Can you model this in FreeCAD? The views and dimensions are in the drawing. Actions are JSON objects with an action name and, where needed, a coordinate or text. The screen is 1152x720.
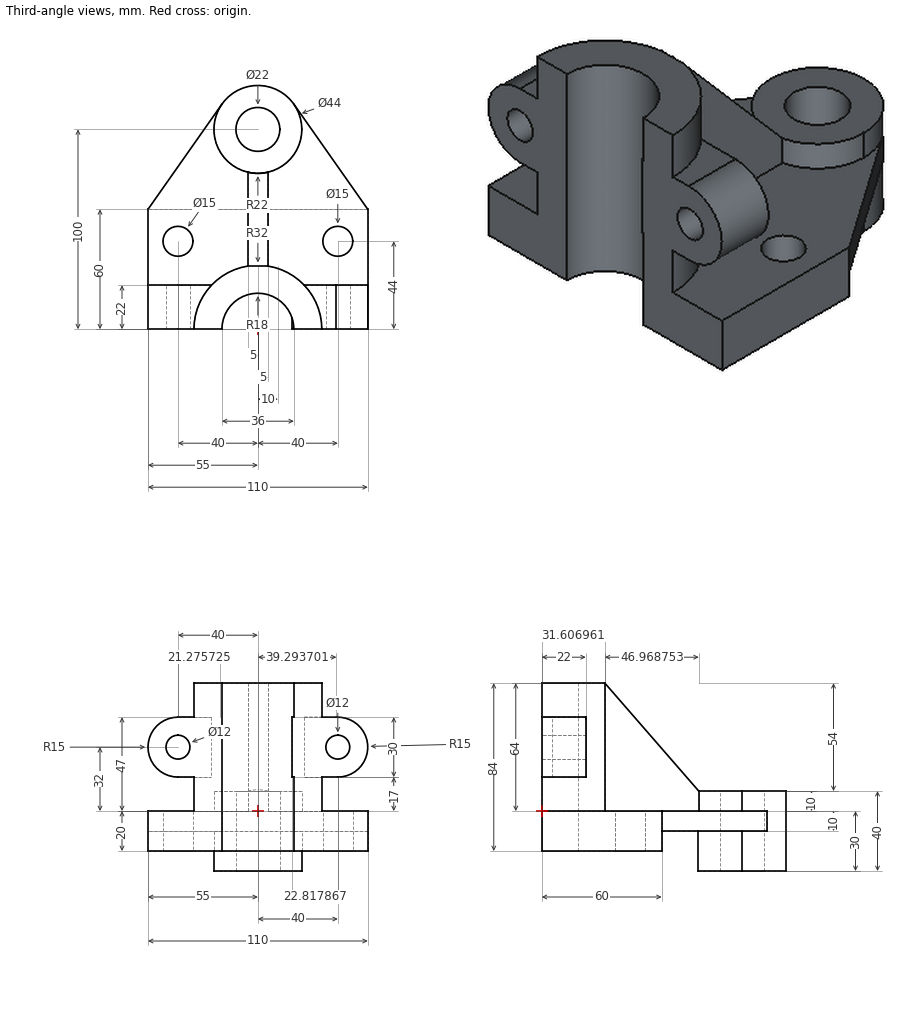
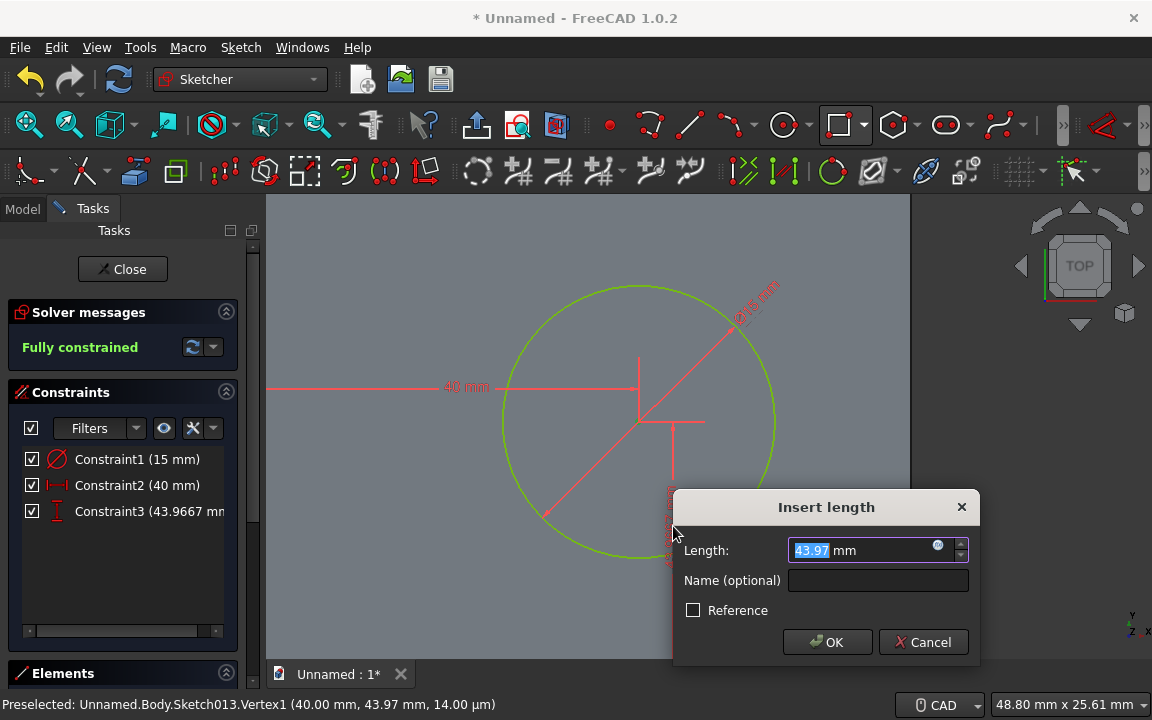
{"action": "type", "text": "44"}
{"action": "key", "text": "Return"}
{"action": "key", "text": "Escape"}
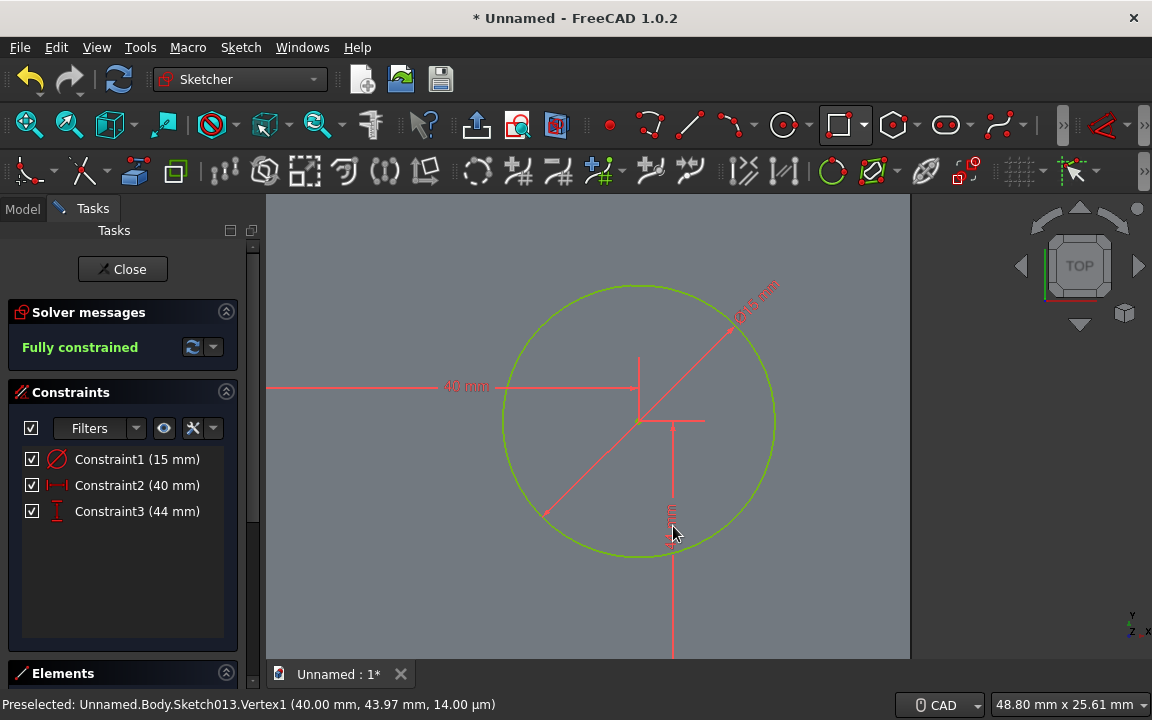
{"action": "left_click", "coordinate": [123, 269]}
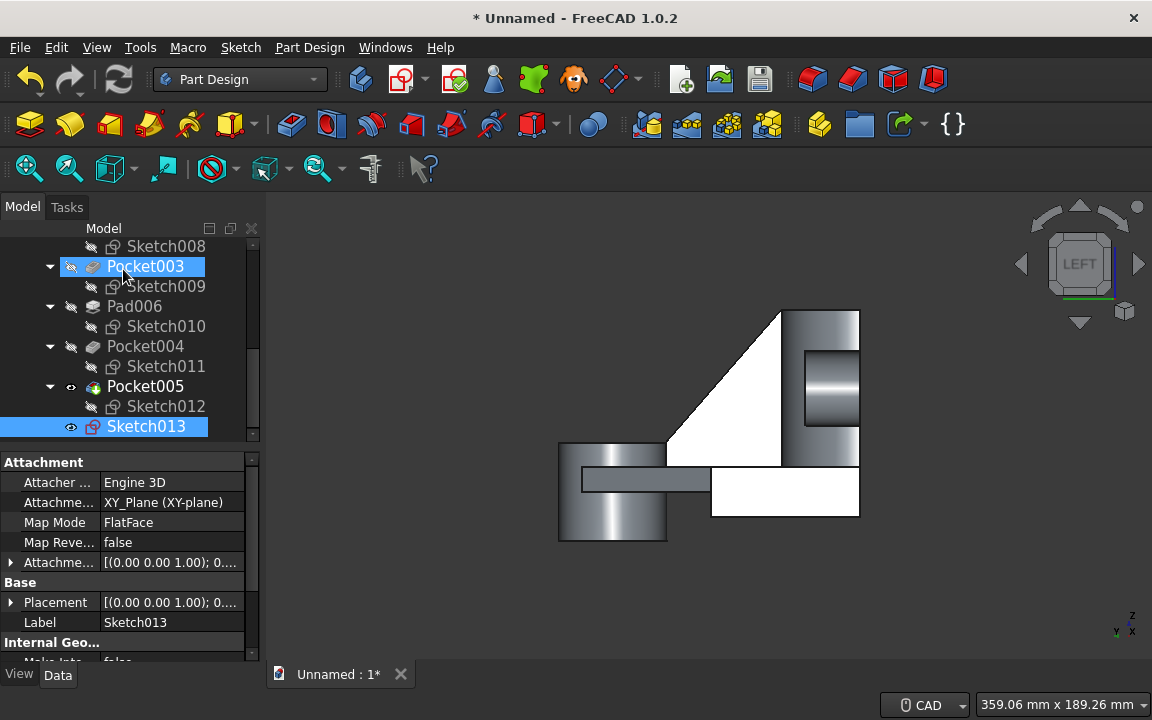
{"action": "left_click", "coordinate": [292, 124]}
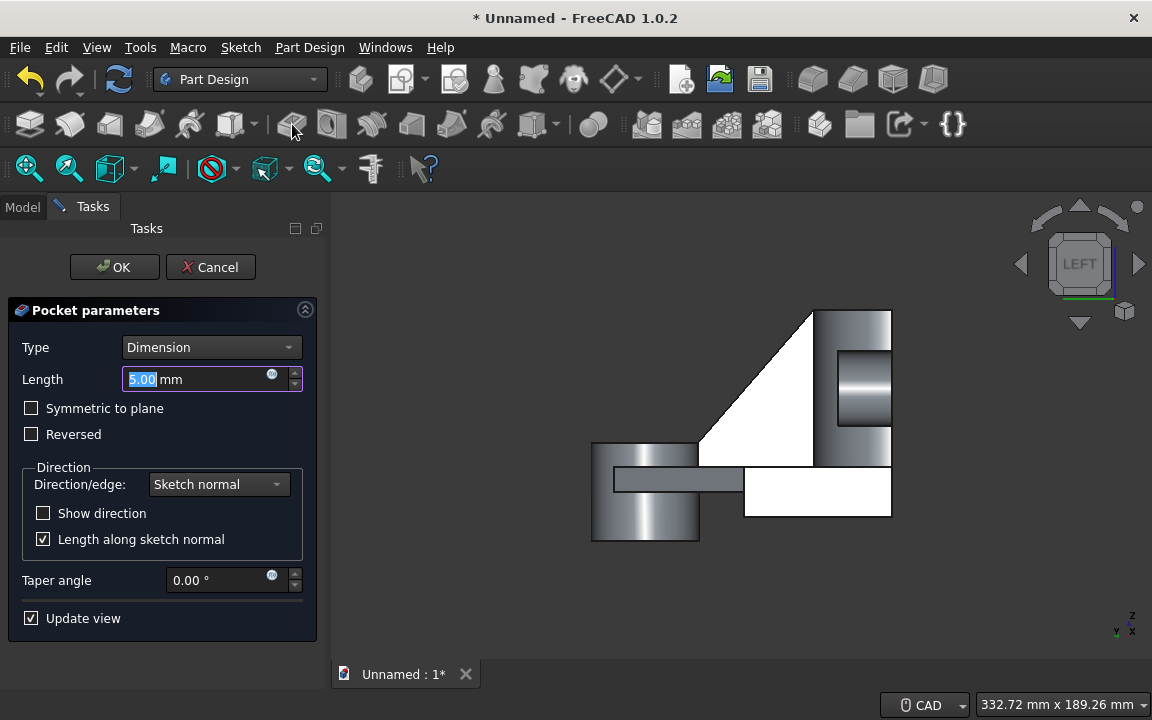
{"action": "type", "text": "20"}
{"action": "key", "text": "Tab"}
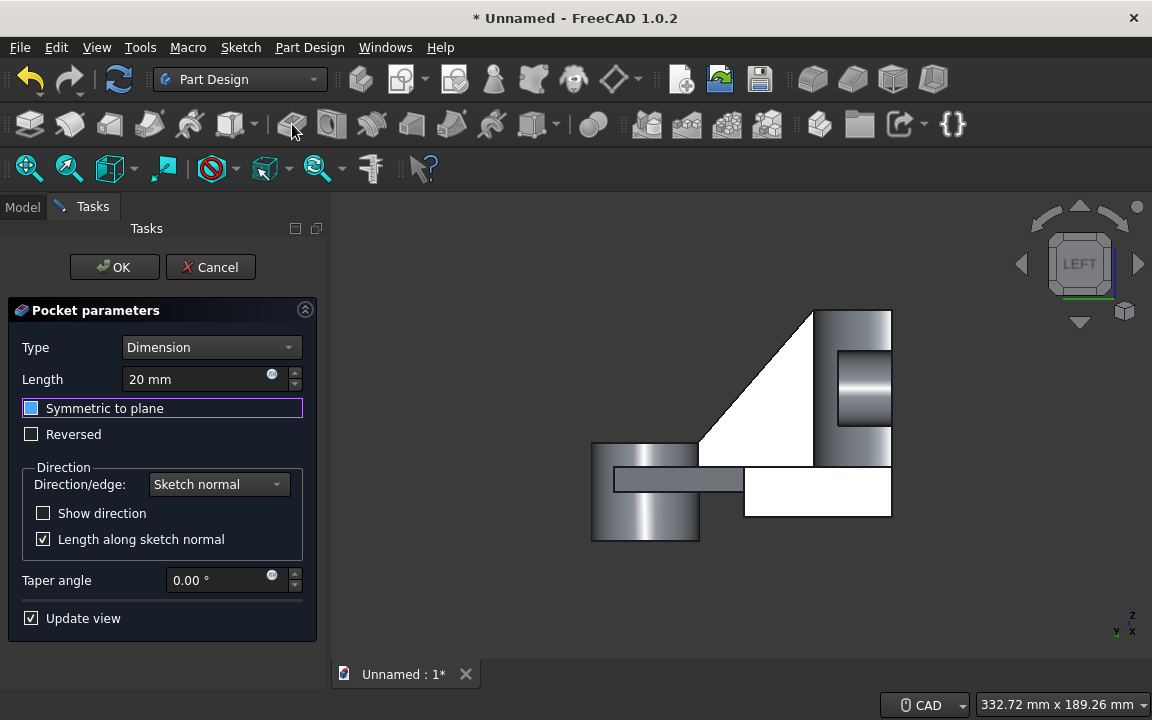
{"action": "left_click", "coordinate": [115, 267]}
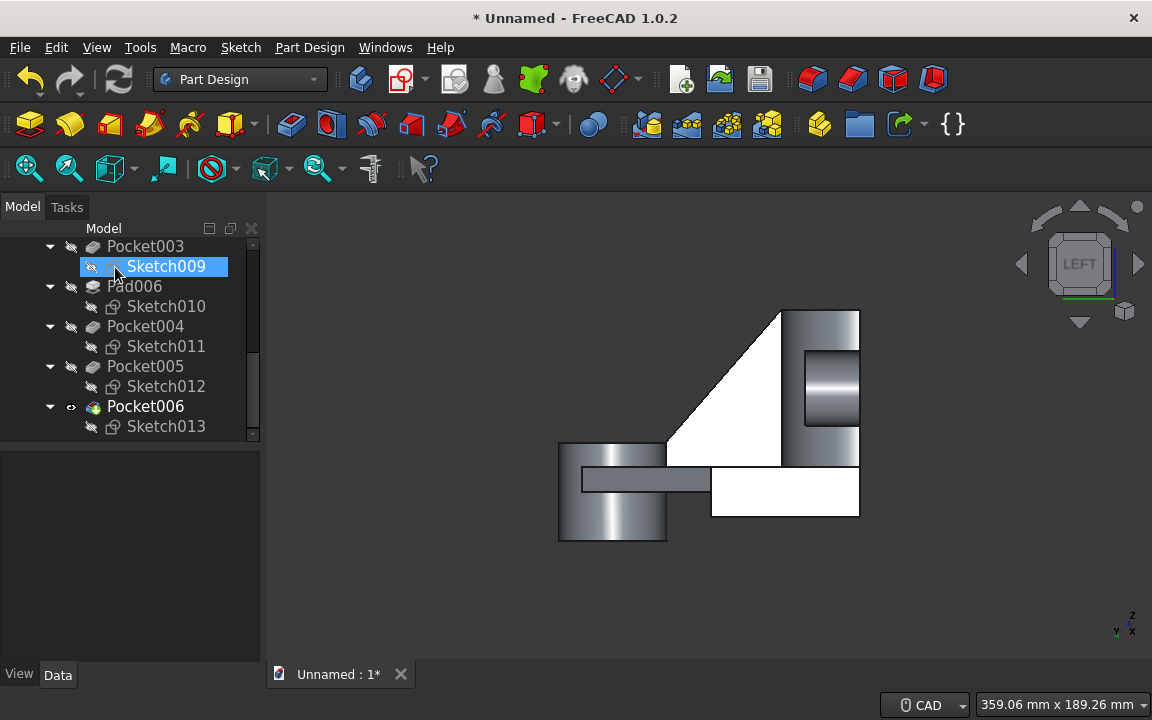
{"action": "key", "text": "0"}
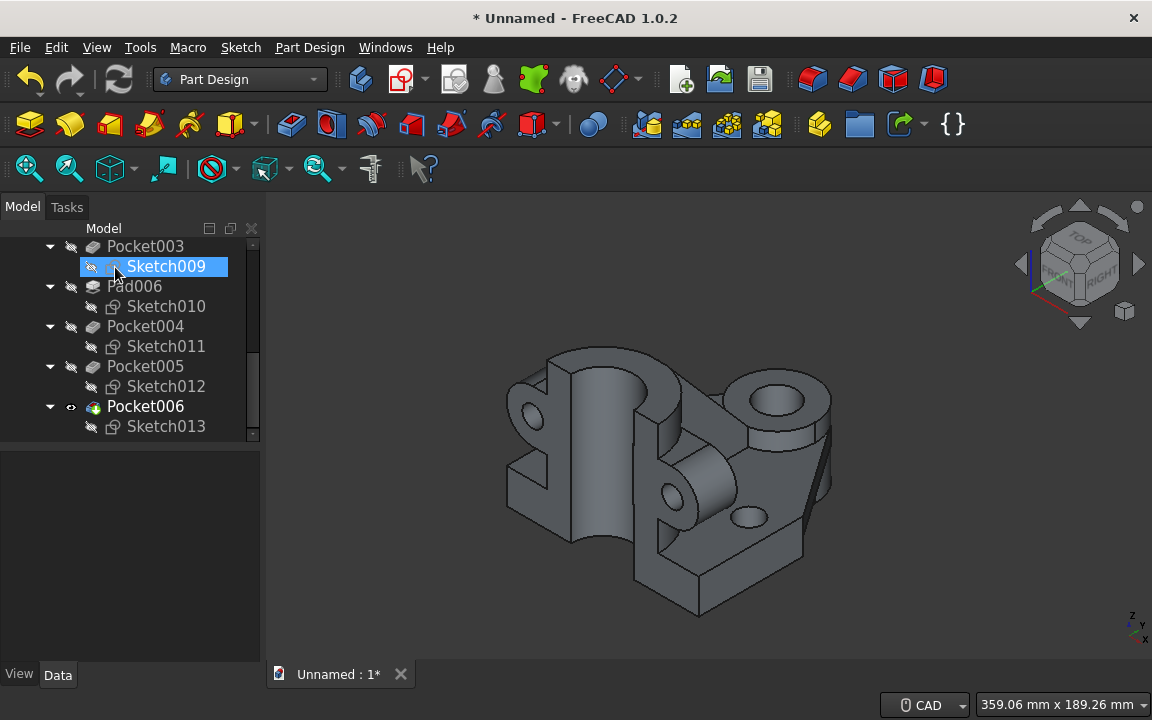
{"action": "key", "text": "2"}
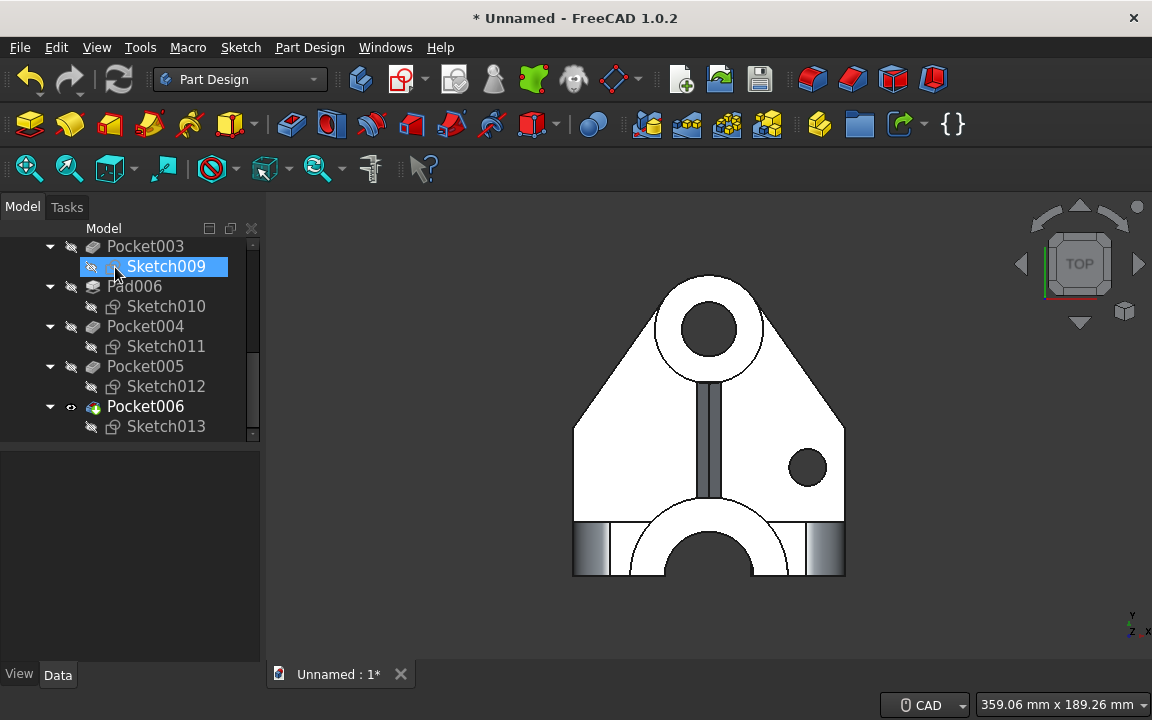
{"action": "left_click", "coordinate": [635, 436]}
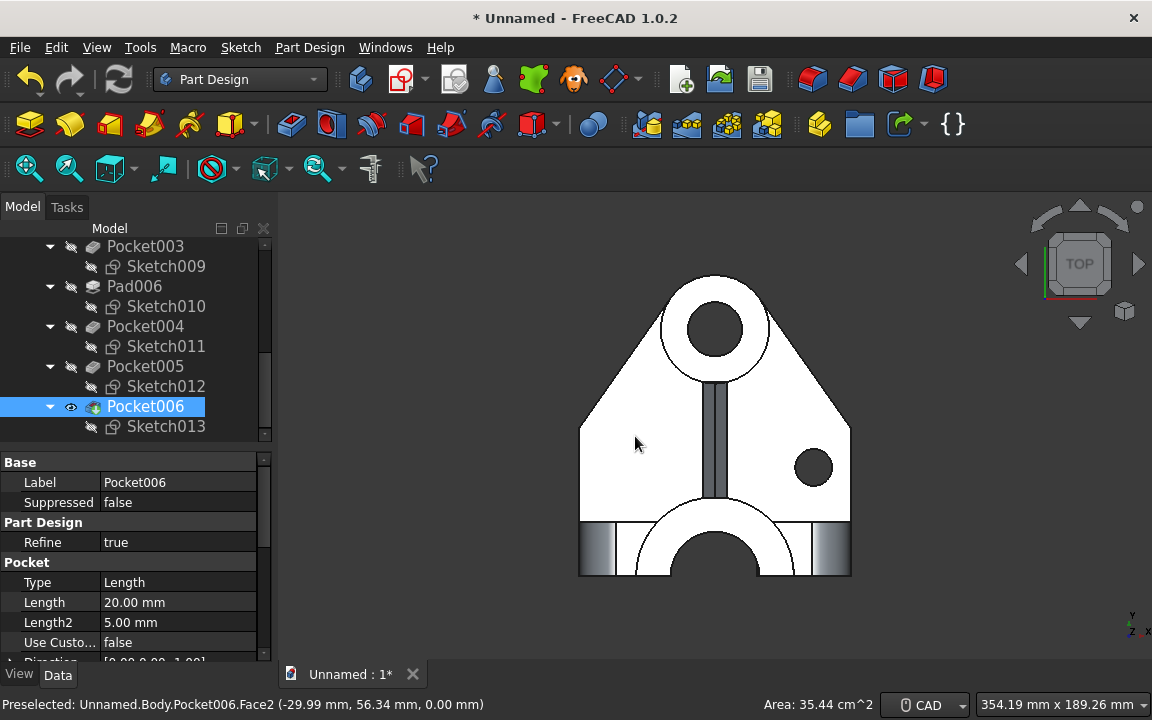
{"action": "left_click", "coordinate": [402, 80]}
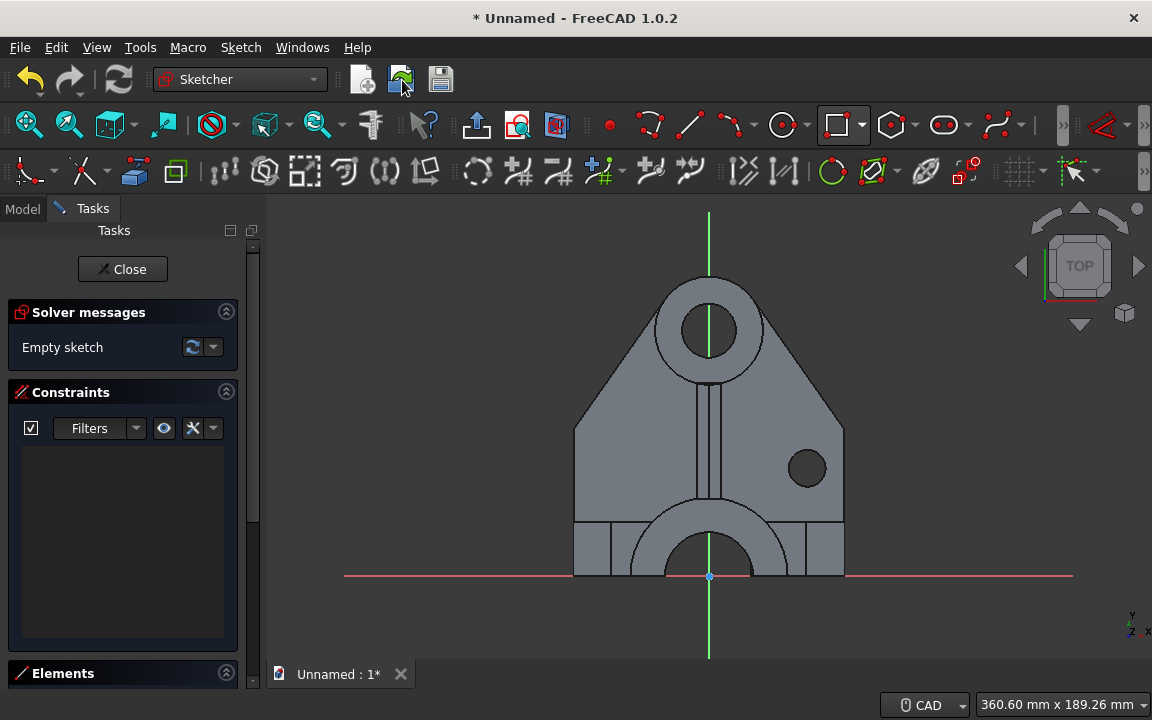
{"action": "left_click", "coordinate": [558, 126]}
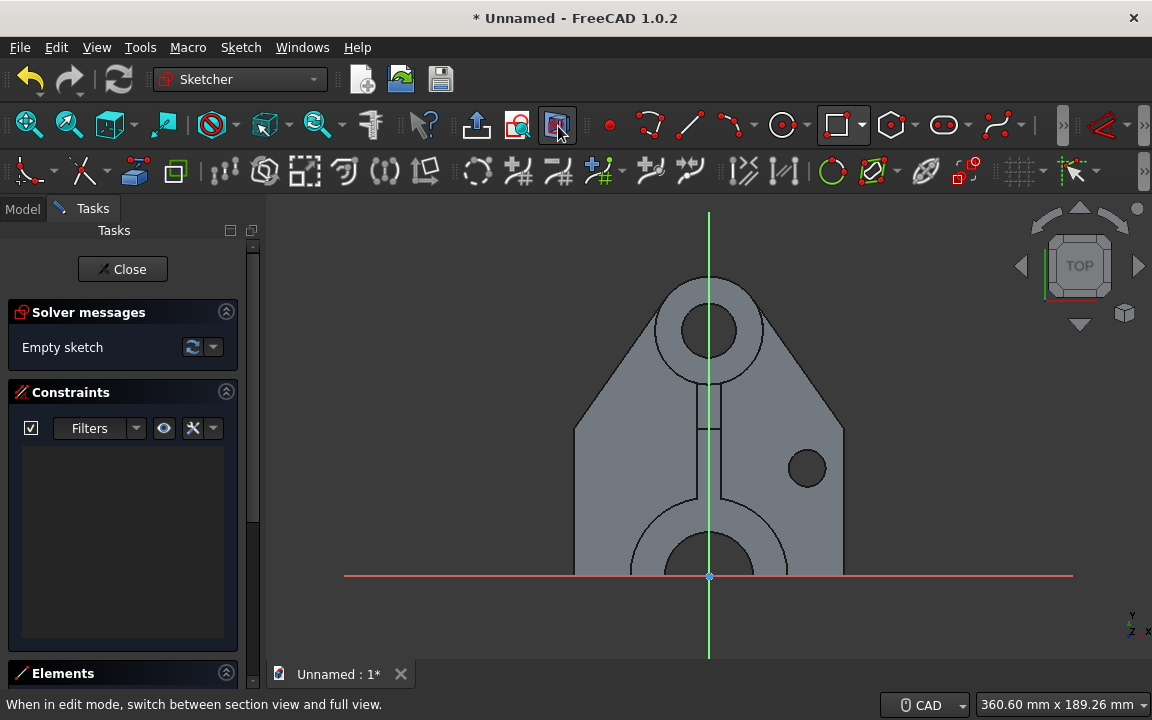
{"action": "scroll", "coordinate": [606, 475], "scroll_direction": "up", "scroll_amount": 10}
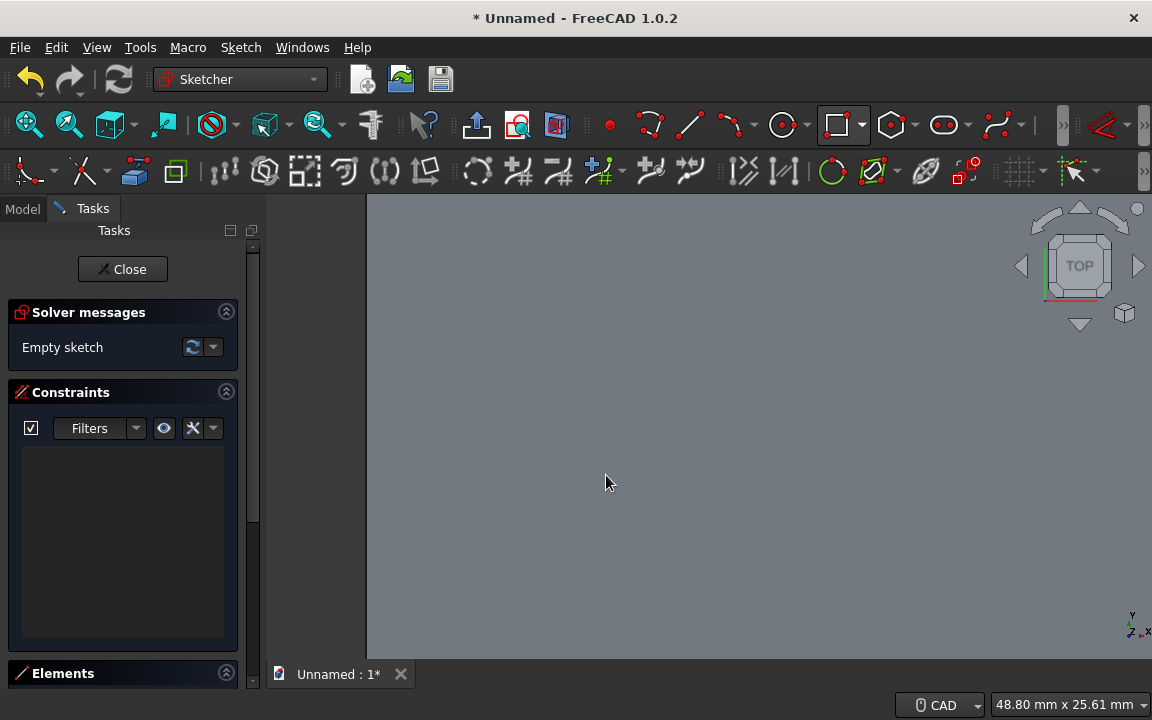
{"action": "left_click", "coordinate": [784, 126]}